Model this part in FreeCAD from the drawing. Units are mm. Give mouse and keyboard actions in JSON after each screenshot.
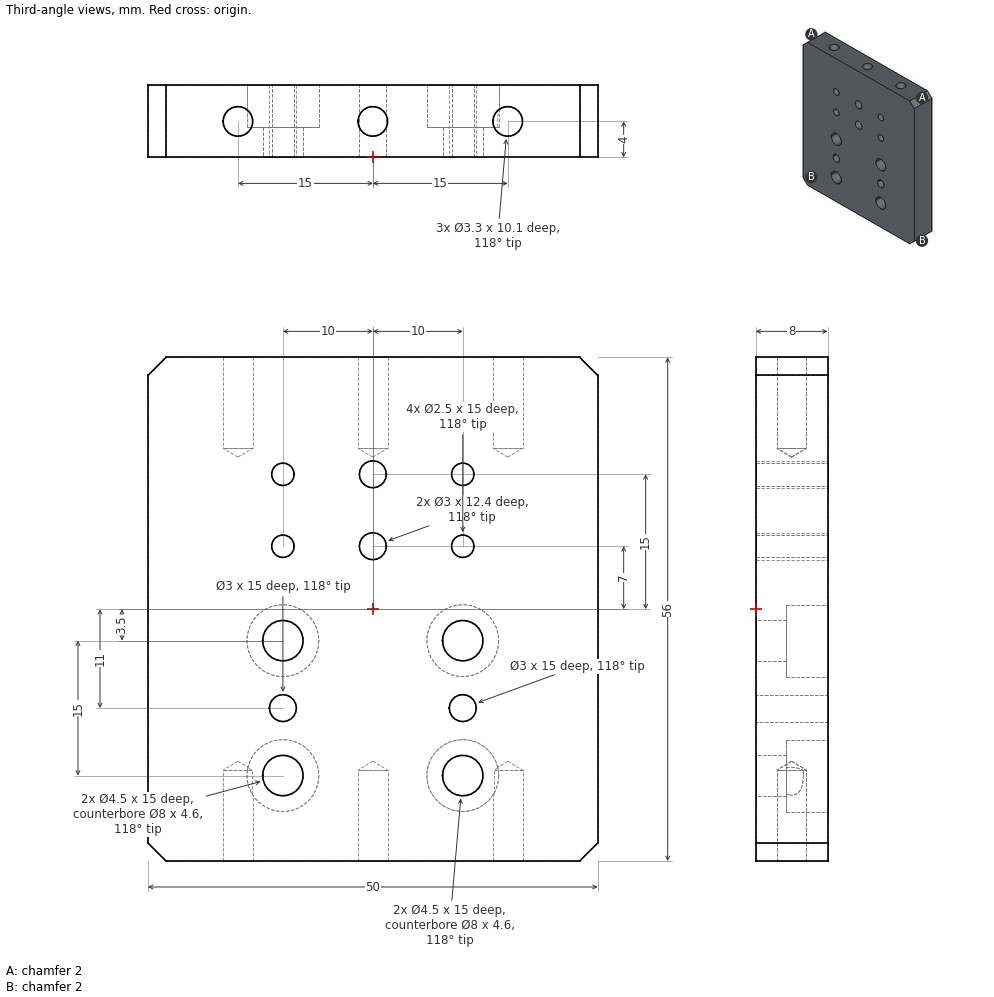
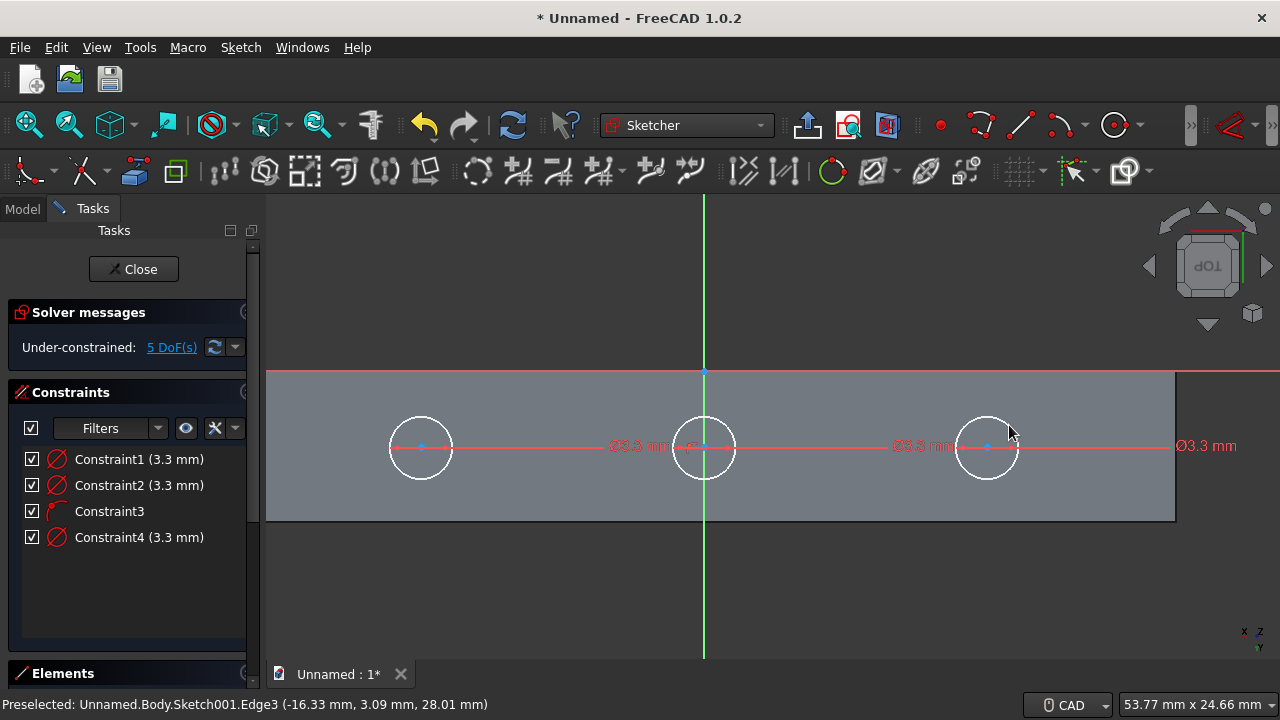
{"action": "left_click", "coordinate": [421, 448]}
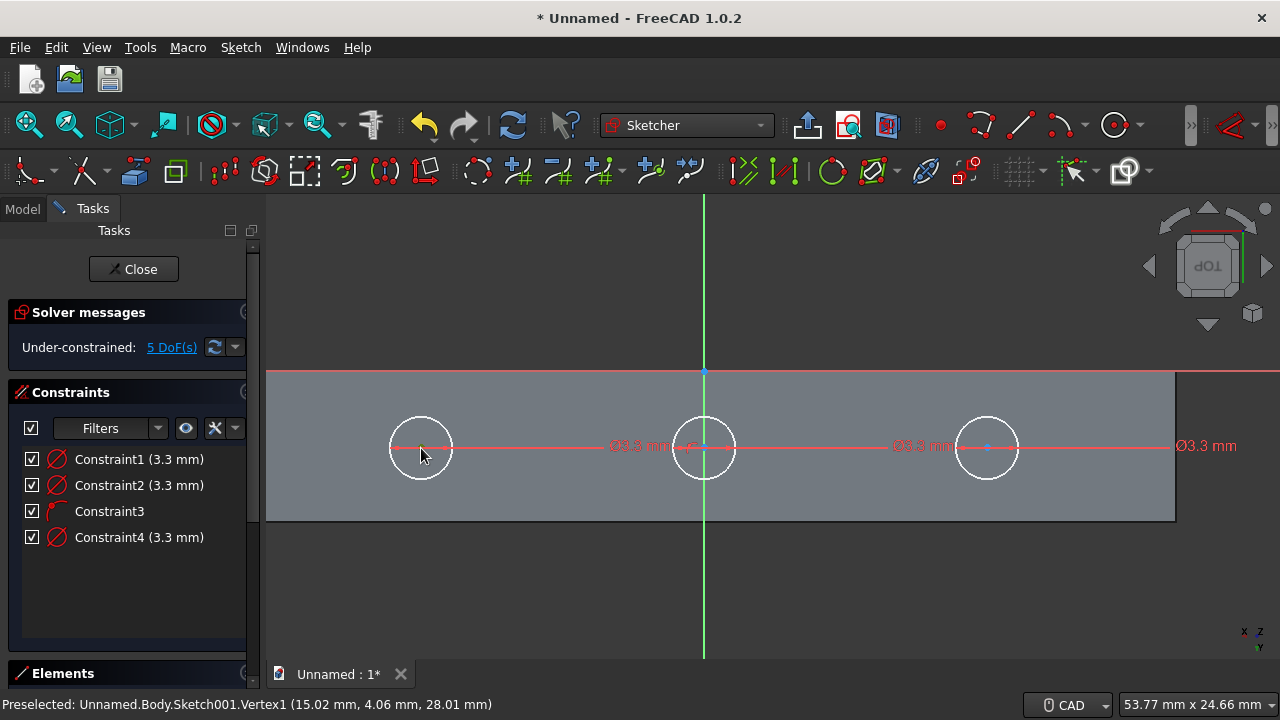
{"action": "left_click", "coordinate": [704, 448]}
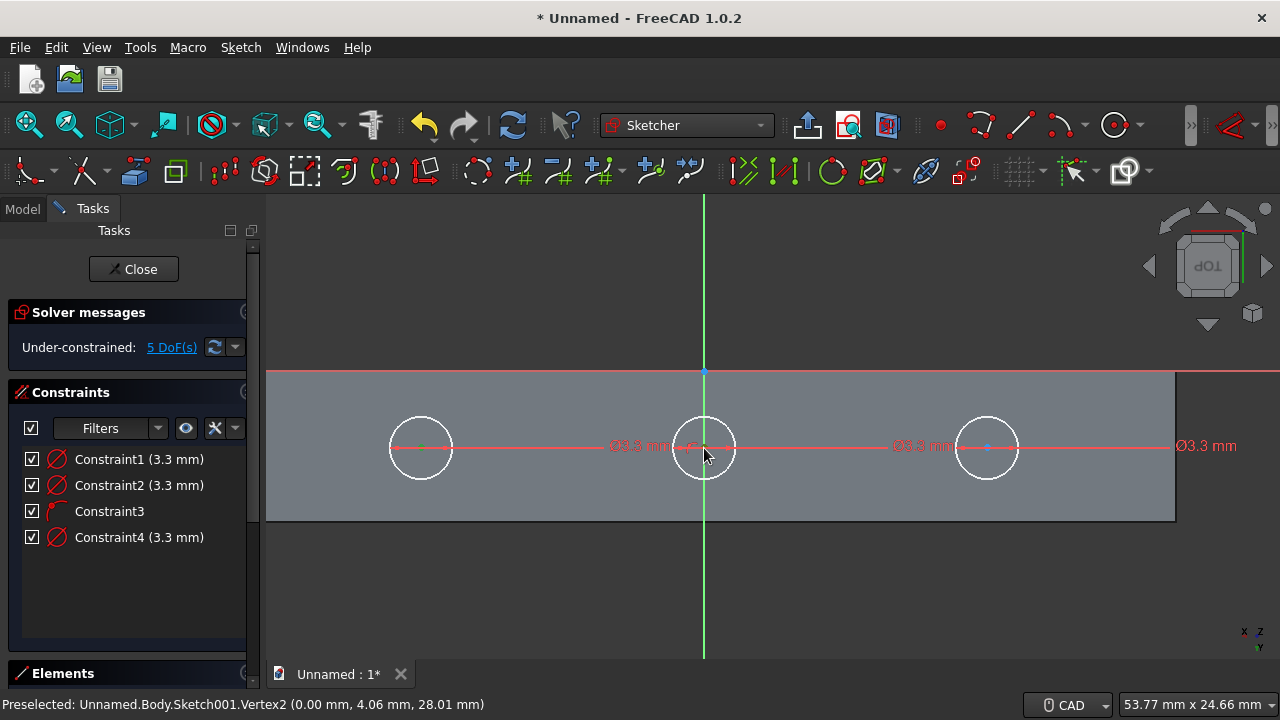
{"action": "key", "text": "h"}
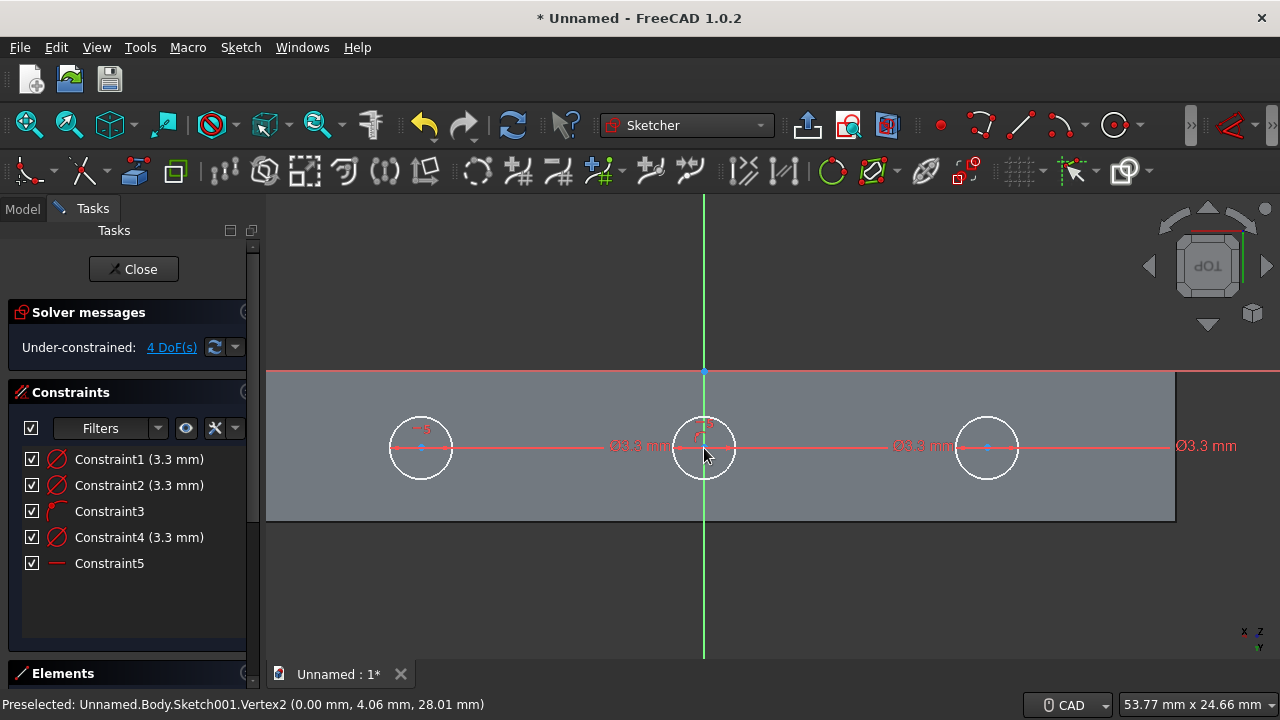
{"action": "left_click", "coordinate": [704, 448]}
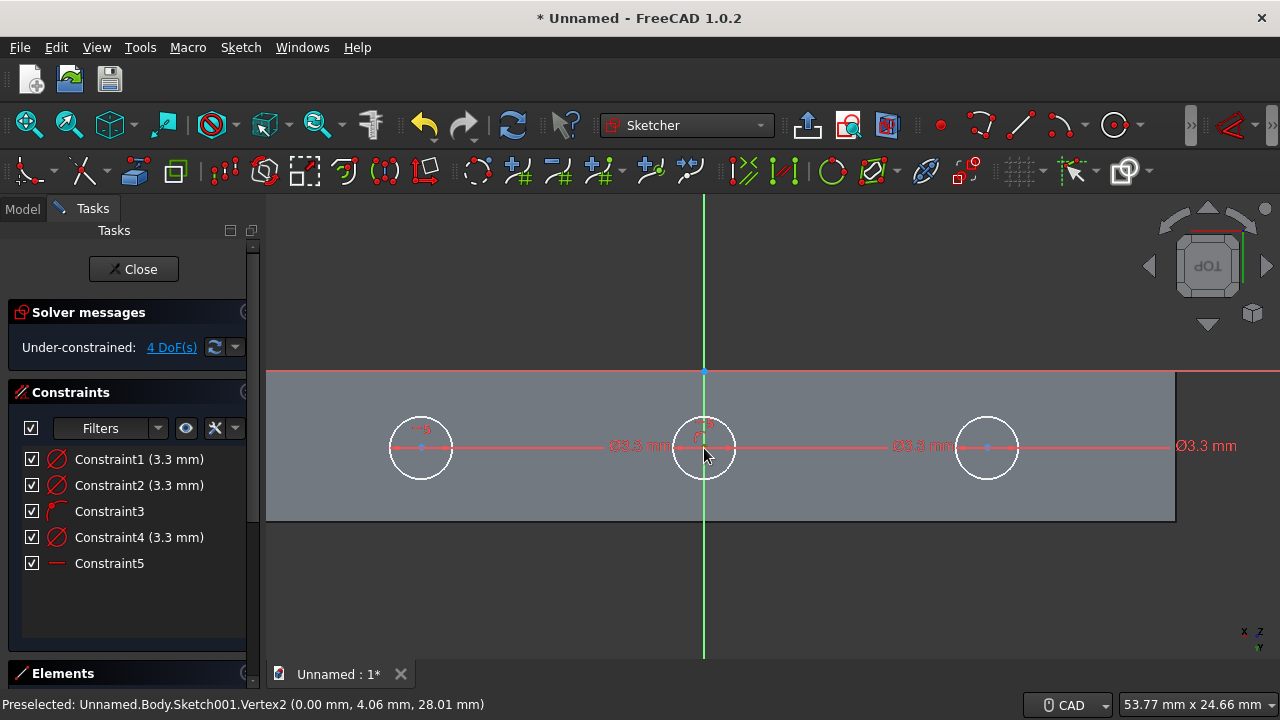
{"action": "left_click", "coordinate": [987, 448]}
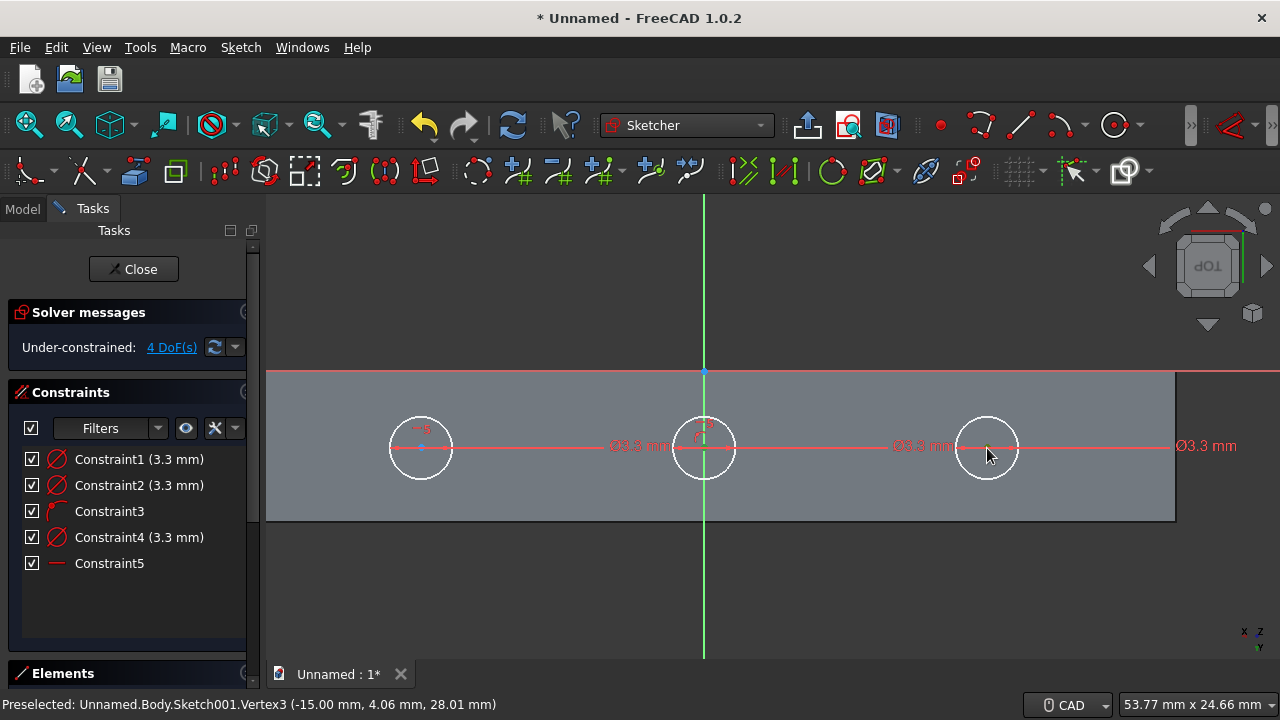
{"action": "key", "text": "h"}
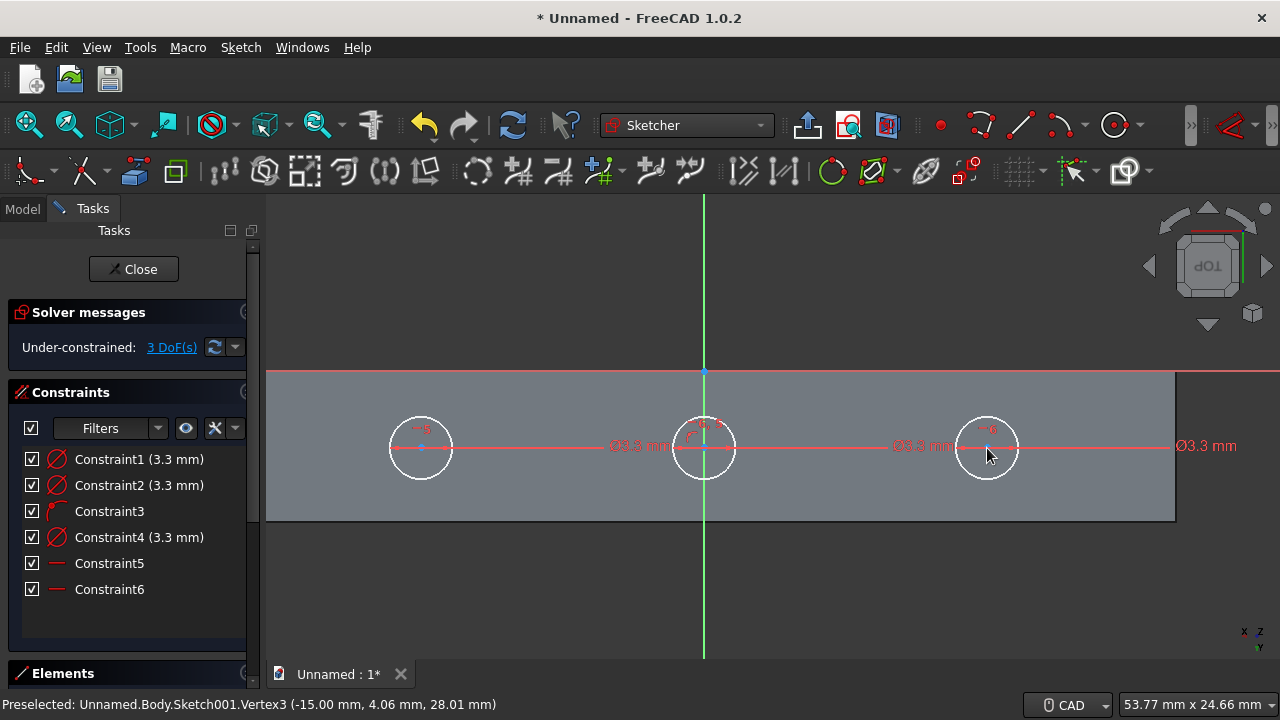
{"action": "left_click", "coordinate": [1230, 126]}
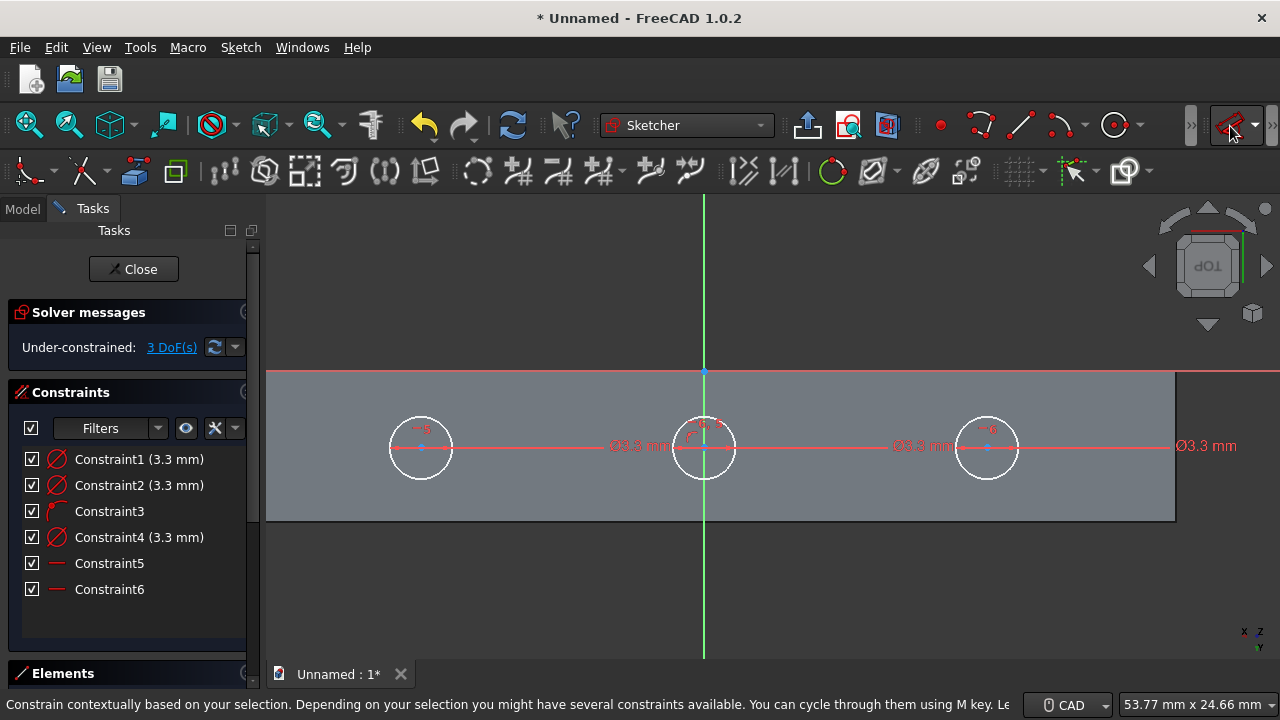
{"action": "left_click", "coordinate": [421, 448]}
{"action": "left_click", "coordinate": [387, 410]}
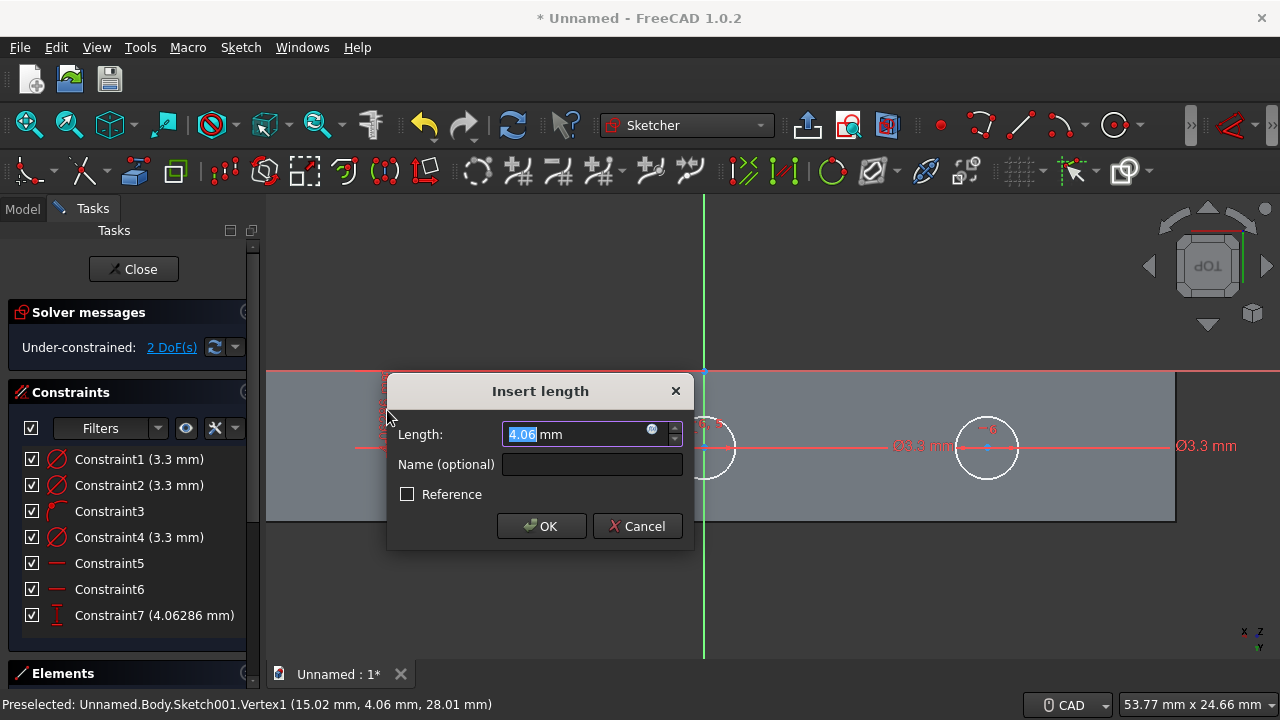
{"action": "type", "text": "4"}
{"action": "key", "text": "Return"}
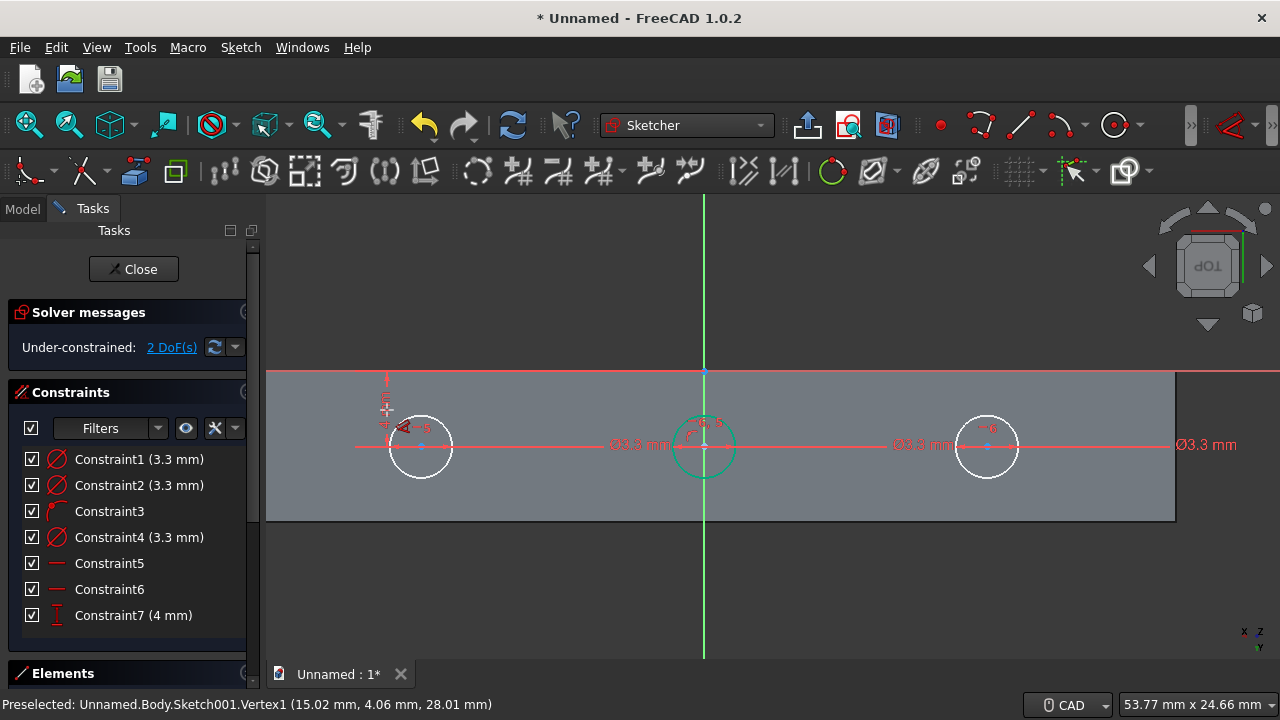
{"action": "left_click", "coordinate": [421, 447]}
{"action": "left_click", "coordinate": [563, 337]}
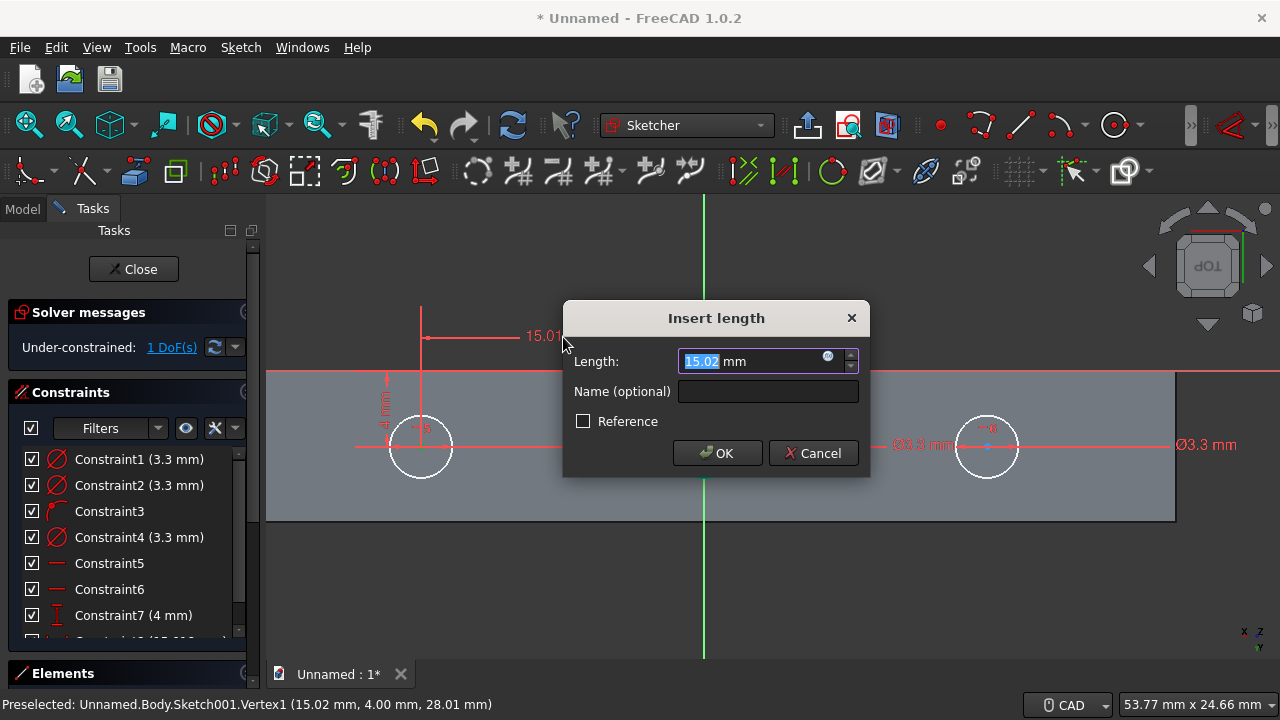
{"action": "type", "text": "15"}
{"action": "key", "text": "Return"}